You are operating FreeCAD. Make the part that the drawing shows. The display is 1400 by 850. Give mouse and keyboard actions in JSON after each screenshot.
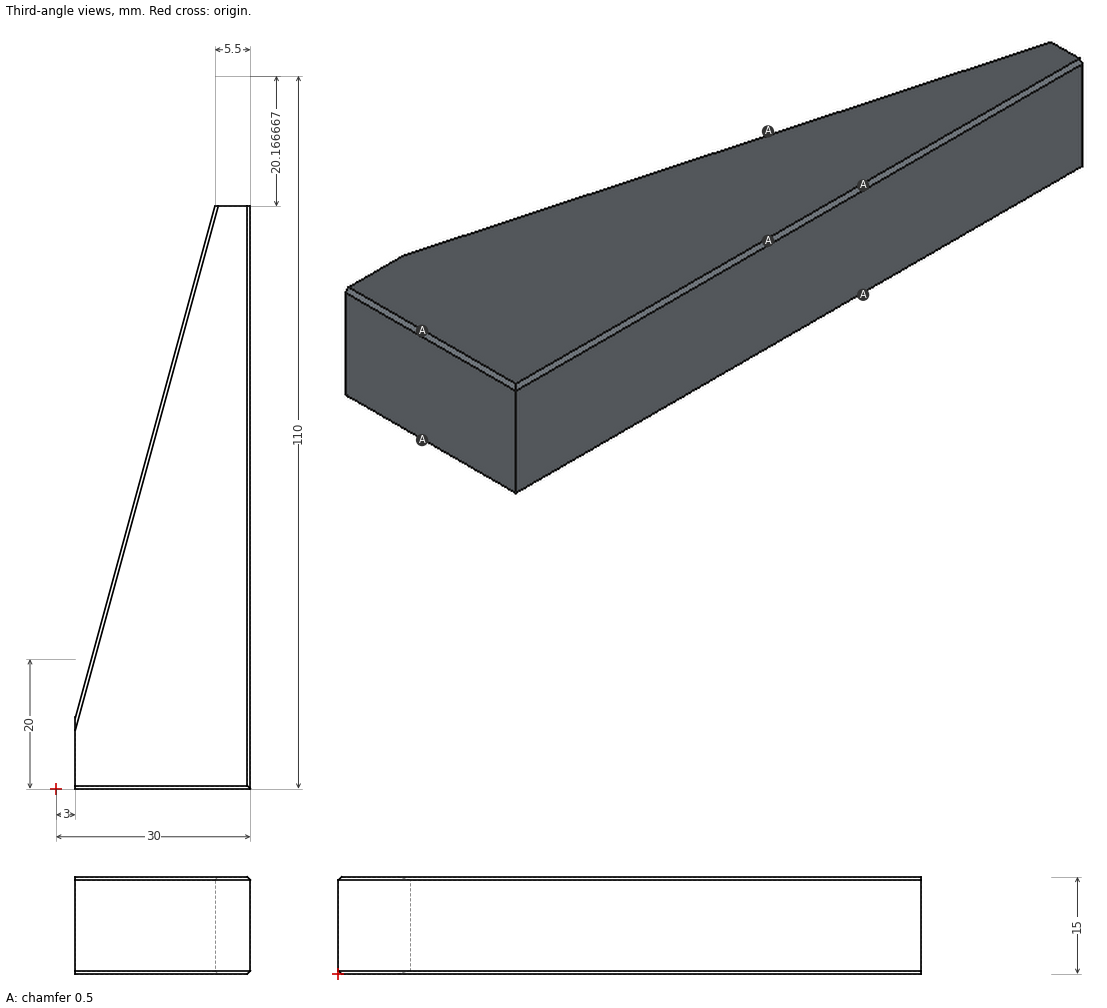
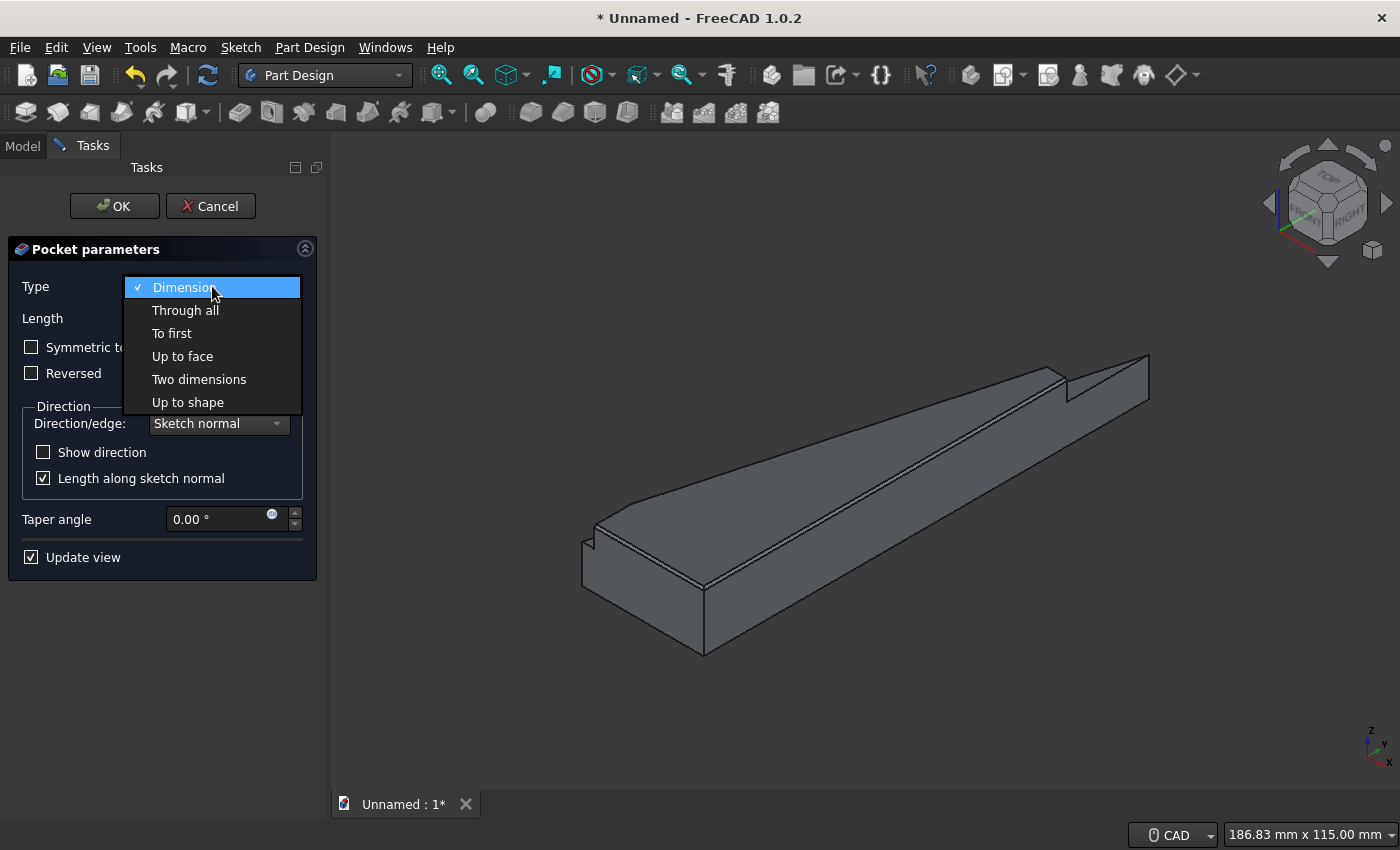
{"action": "left_click", "coordinate": [212, 310]}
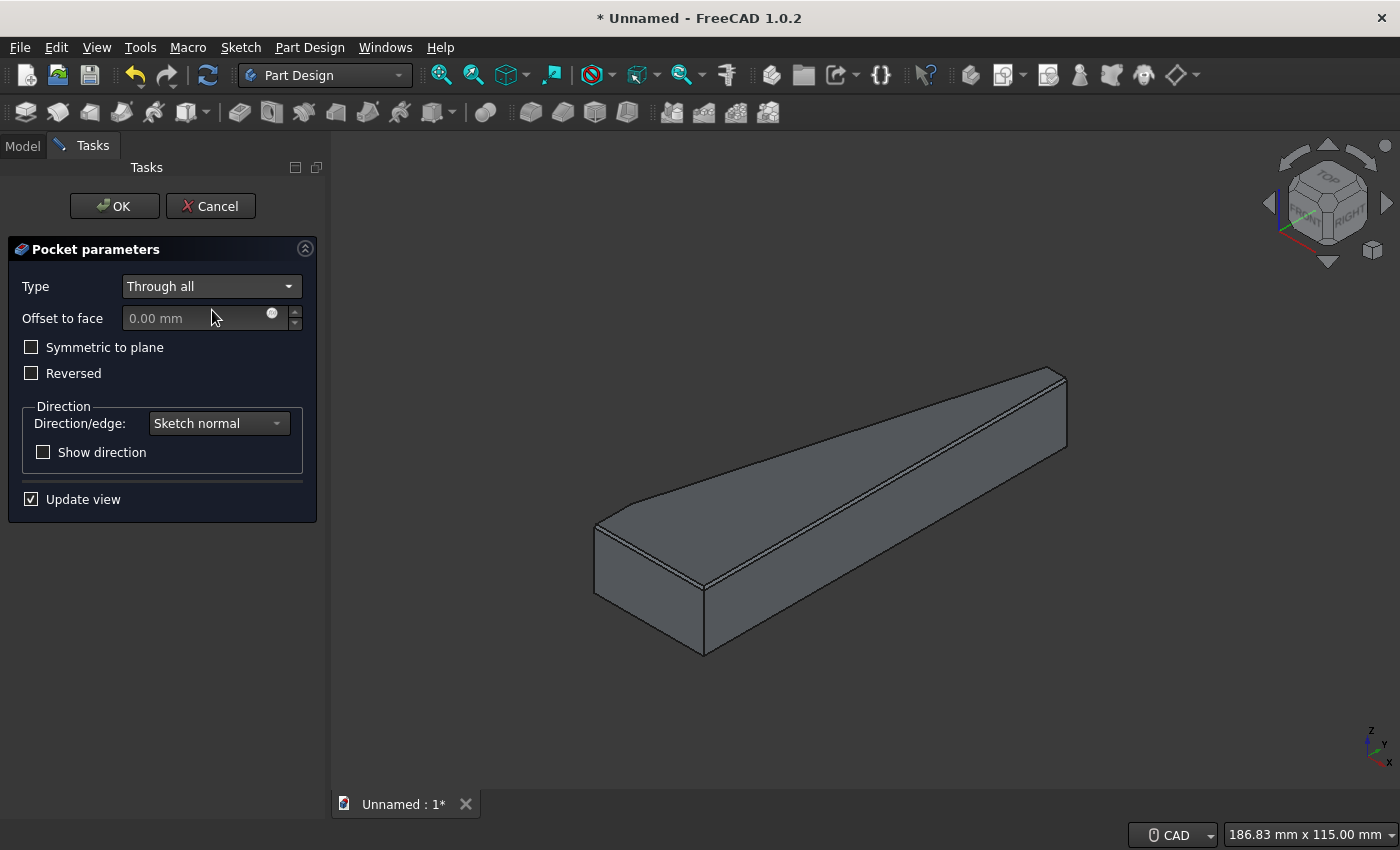
{"action": "left_click", "coordinate": [115, 206]}